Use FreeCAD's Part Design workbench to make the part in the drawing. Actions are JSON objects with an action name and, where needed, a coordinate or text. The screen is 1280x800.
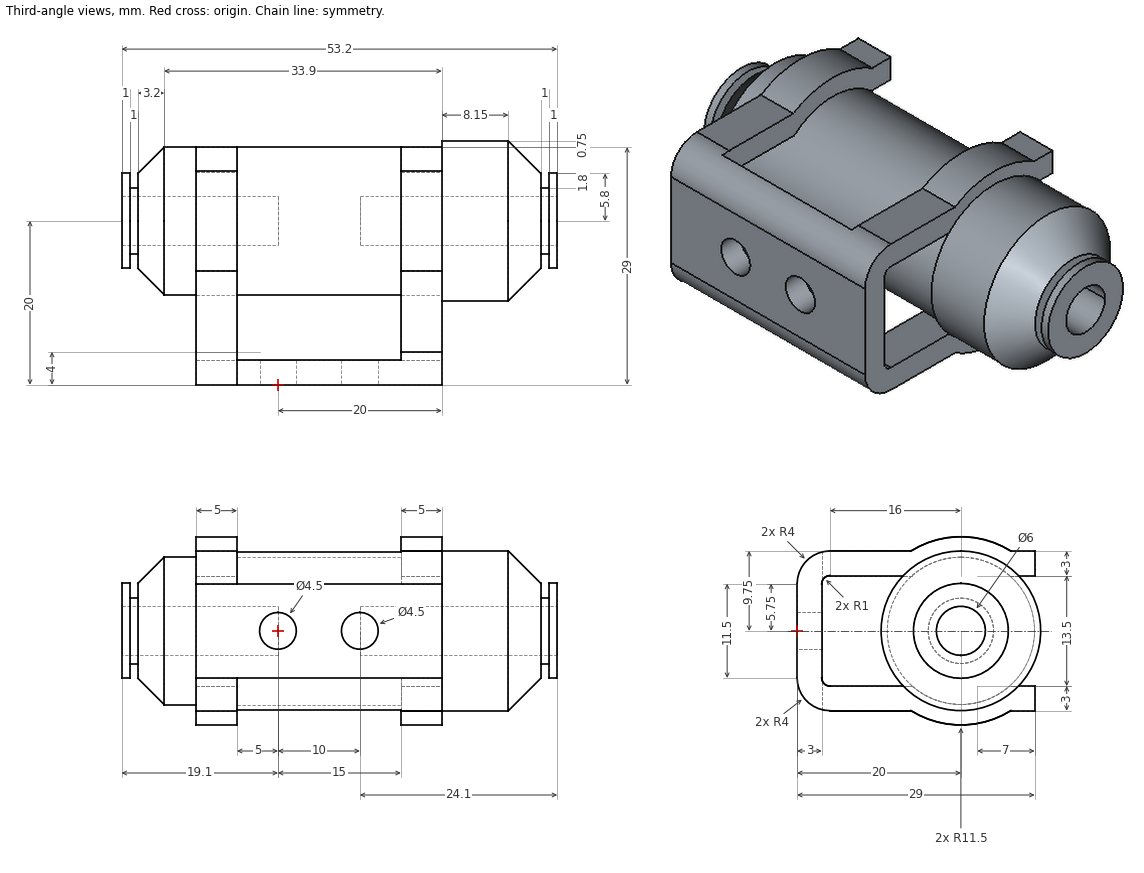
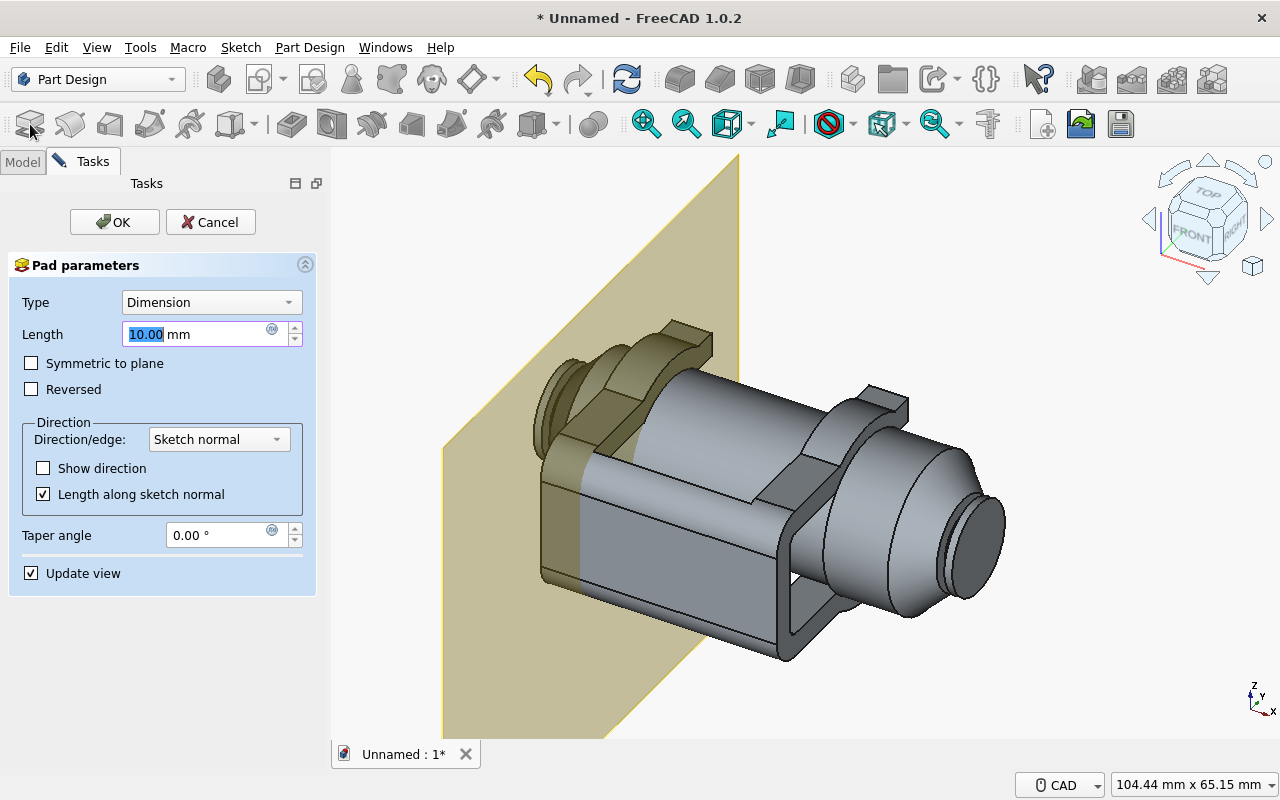
{"action": "type", "text": "5"}
{"action": "key", "text": "Tab"}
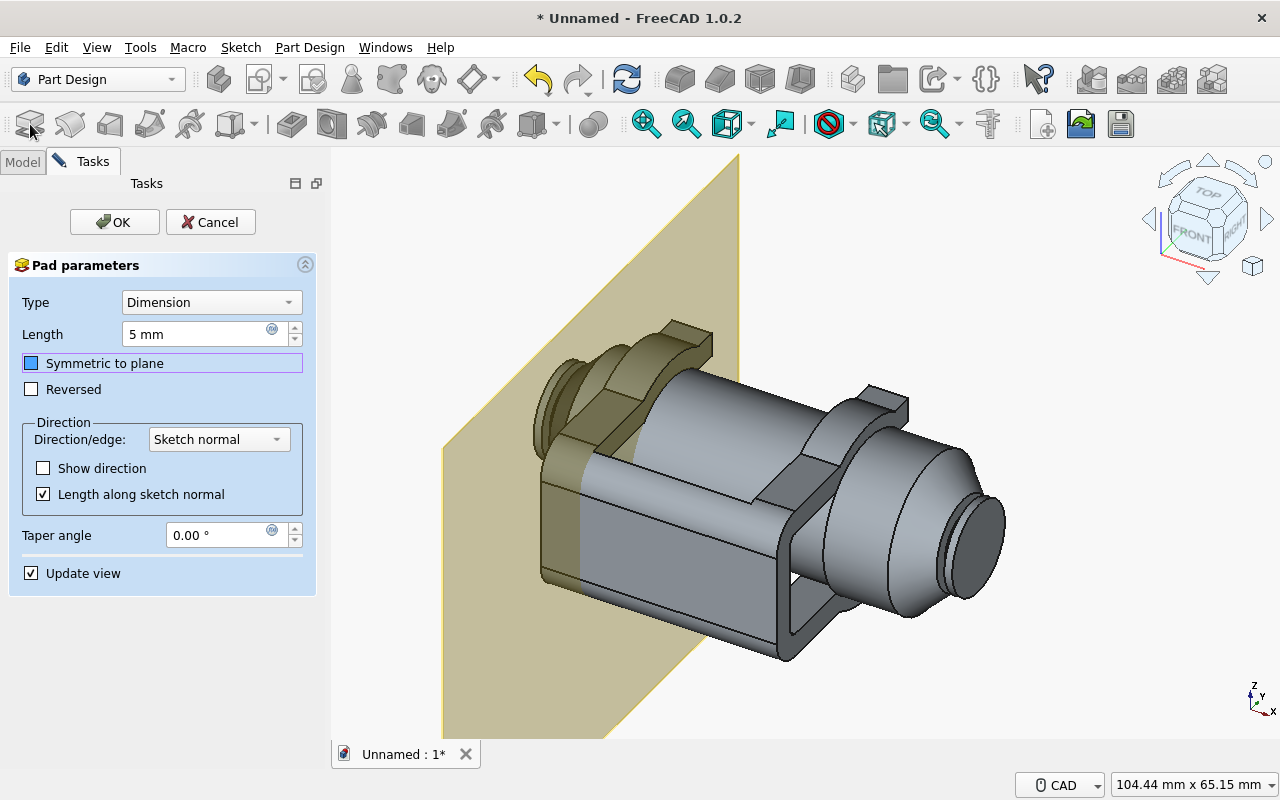
{"action": "left_click", "coordinate": [115, 222]}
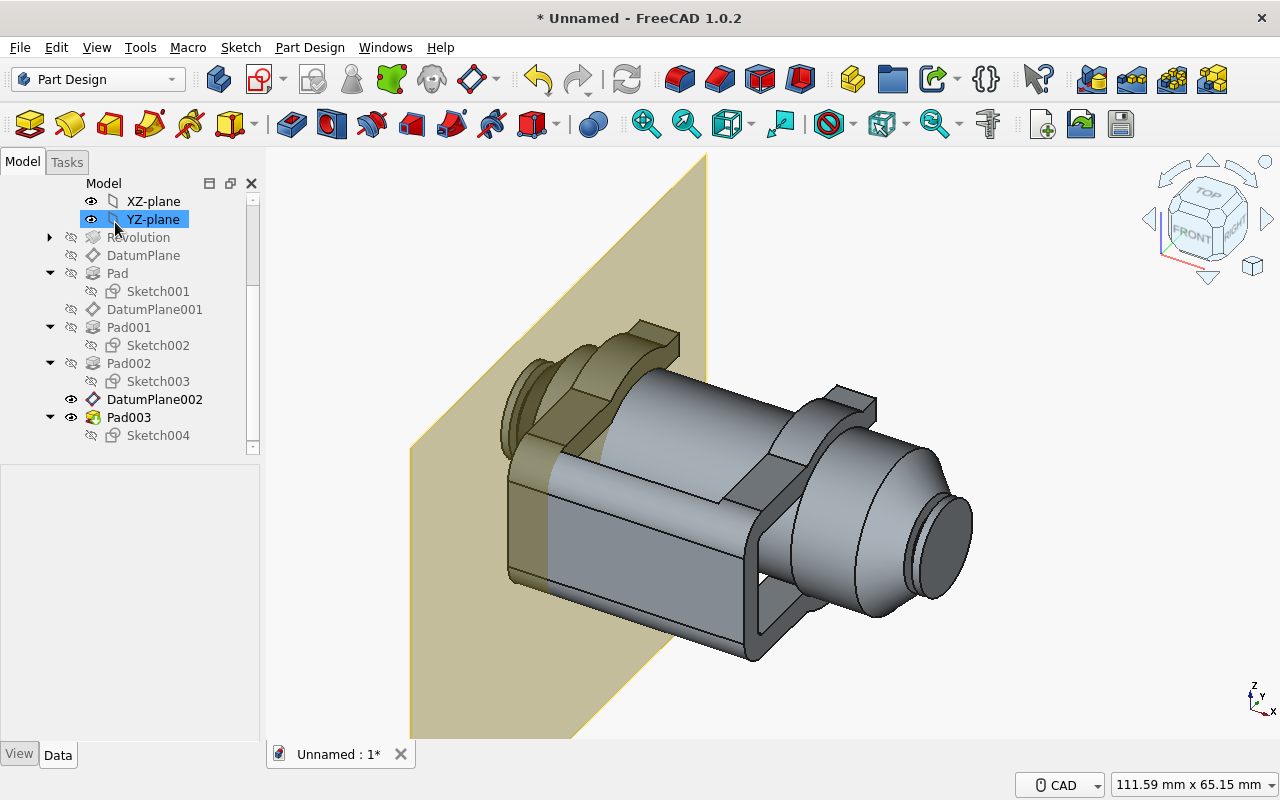
{"action": "left_click", "coordinate": [116, 399]}
{"action": "key", "text": "space"}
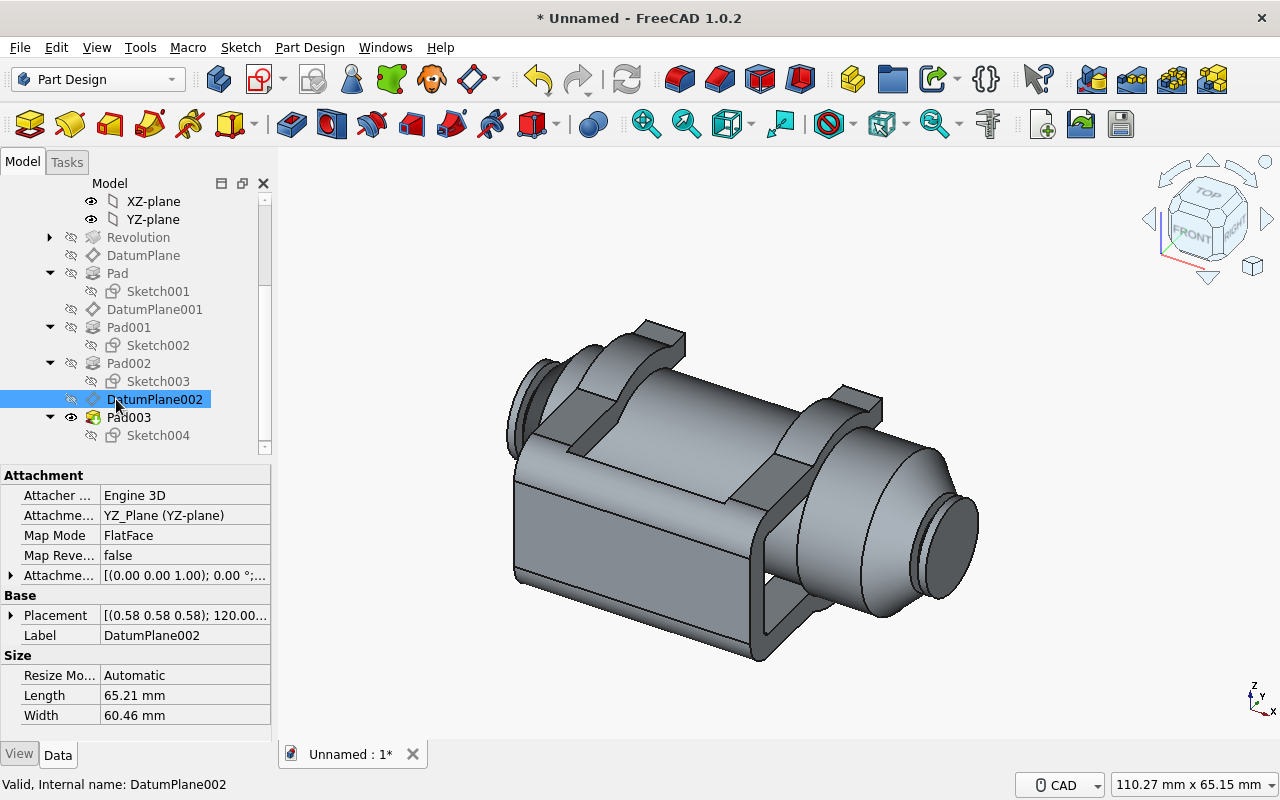
{"action": "left_click", "coordinate": [318, 699]}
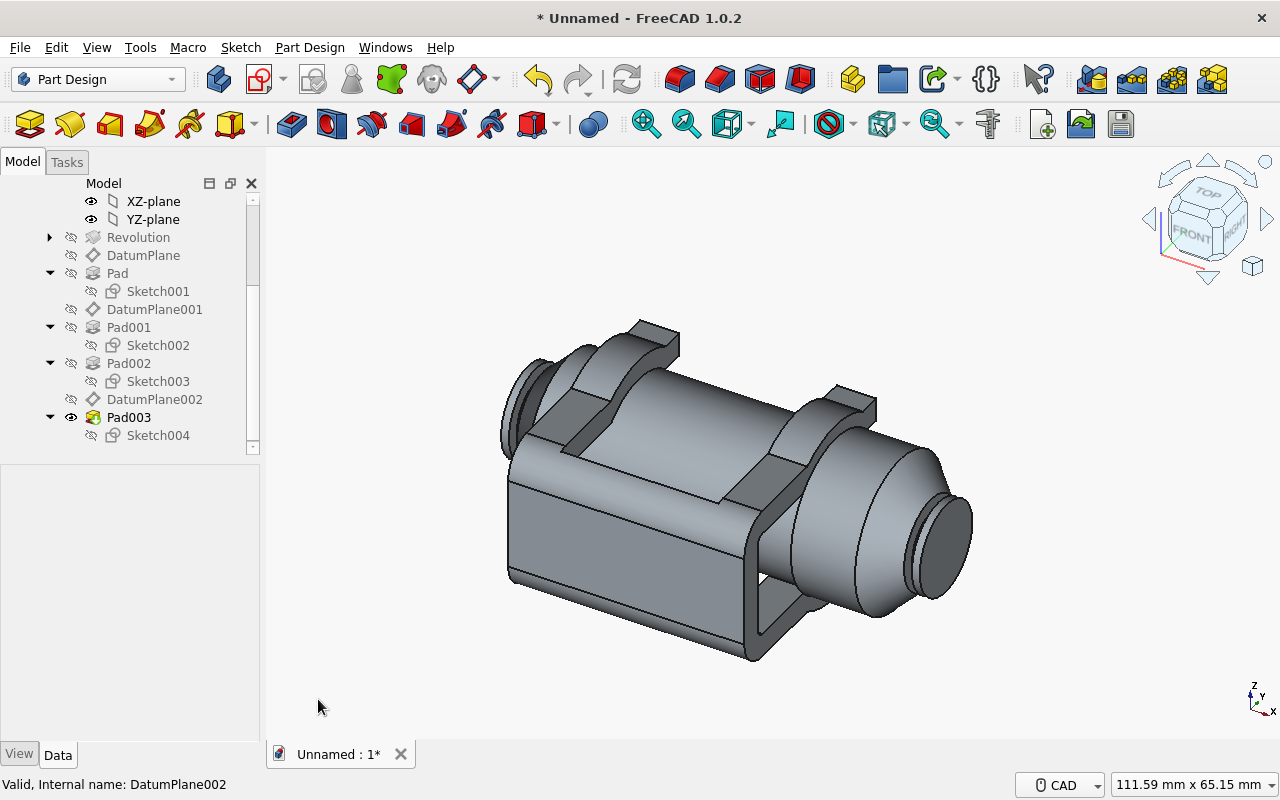
{"action": "left_click", "coordinate": [260, 80]}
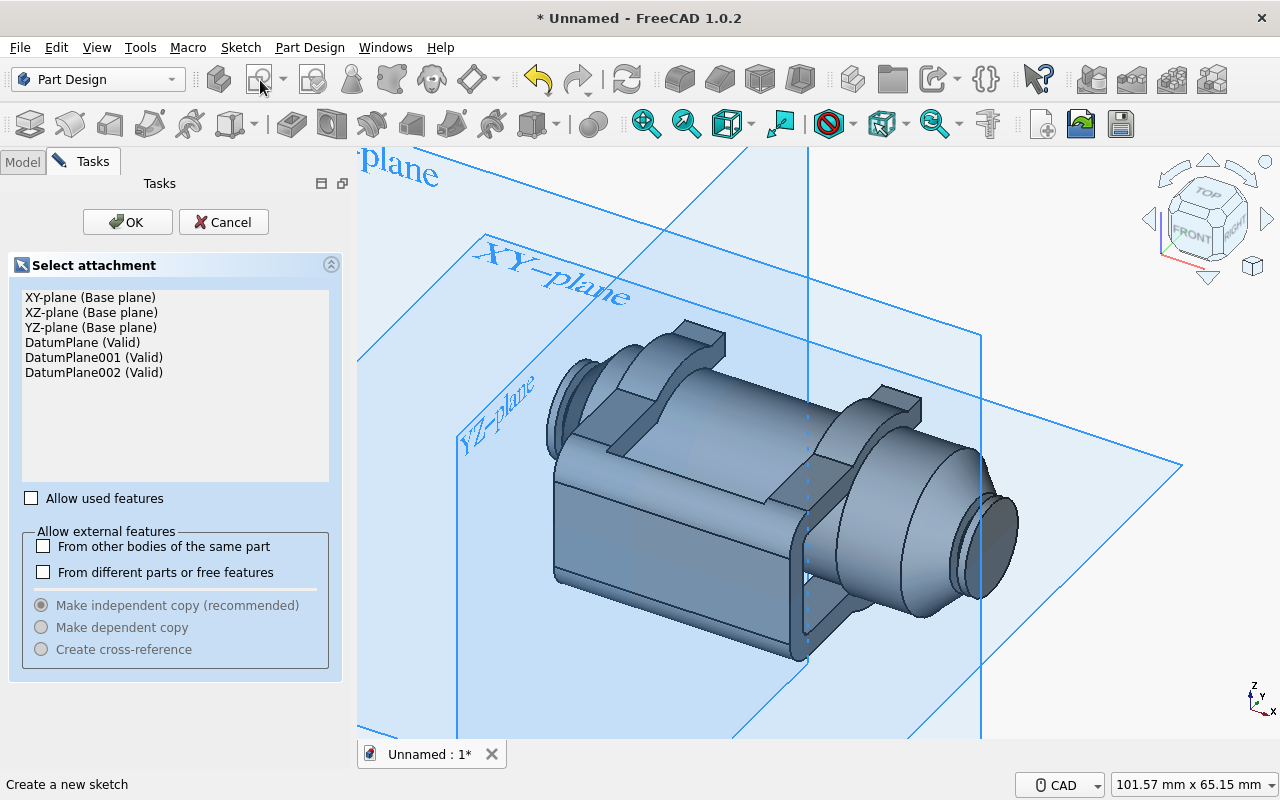
{"action": "left_click", "coordinate": [82, 312]}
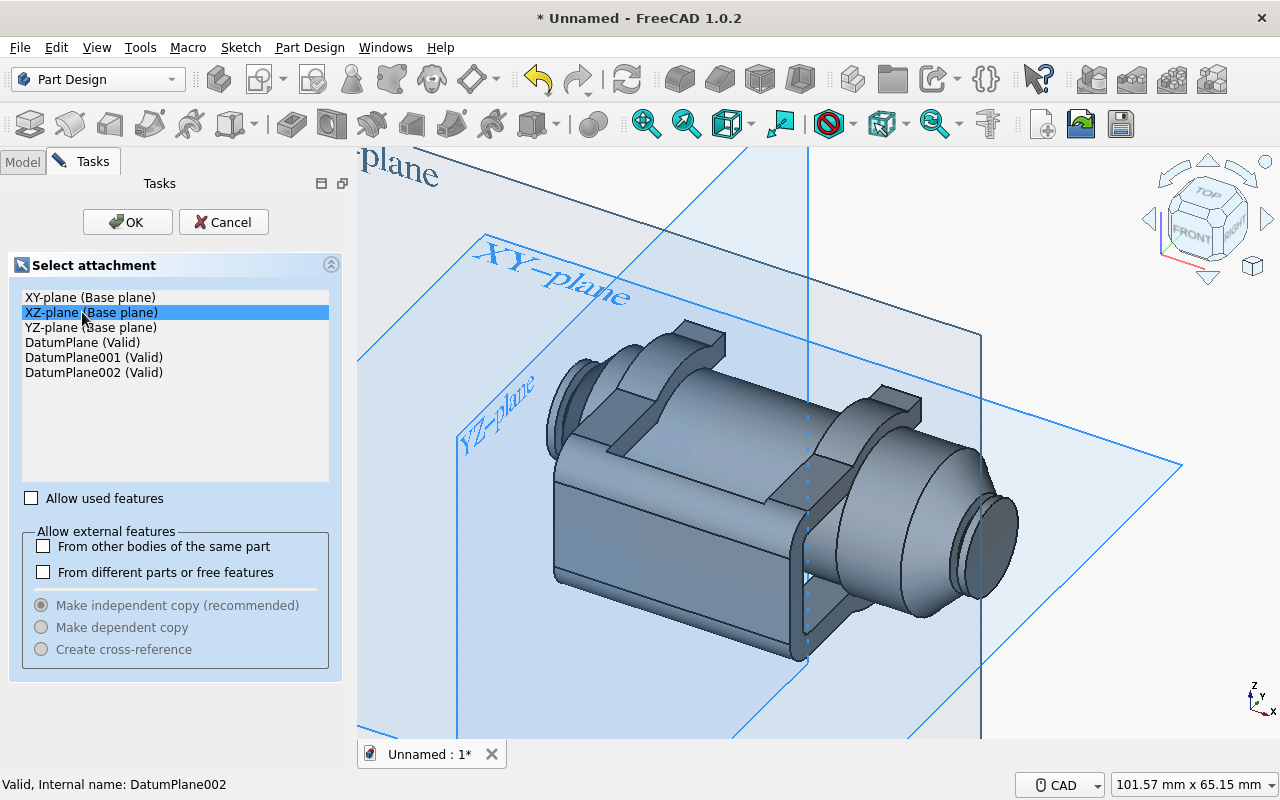
{"action": "left_click", "coordinate": [128, 222]}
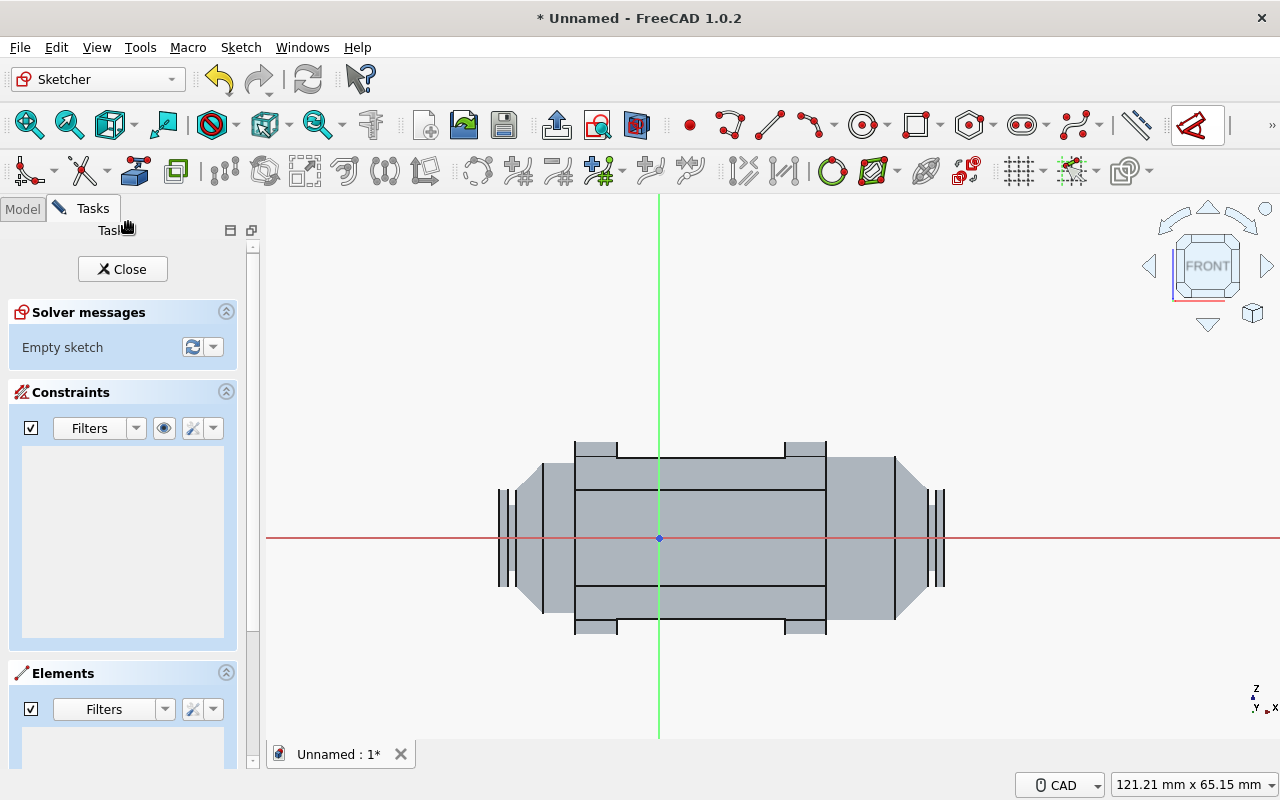
{"action": "scroll", "coordinate": [653, 547], "scroll_direction": "up", "scroll_amount": 11}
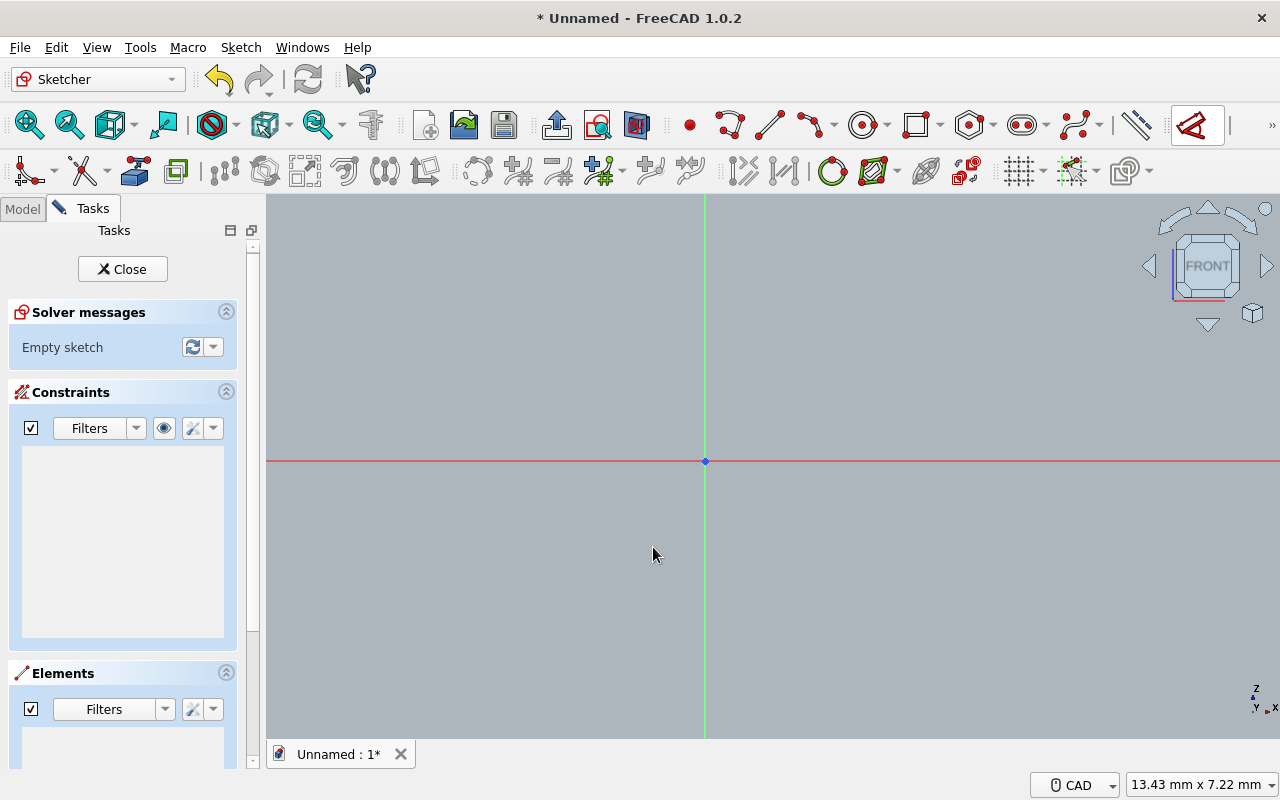
{"action": "left_click", "coordinate": [864, 126]}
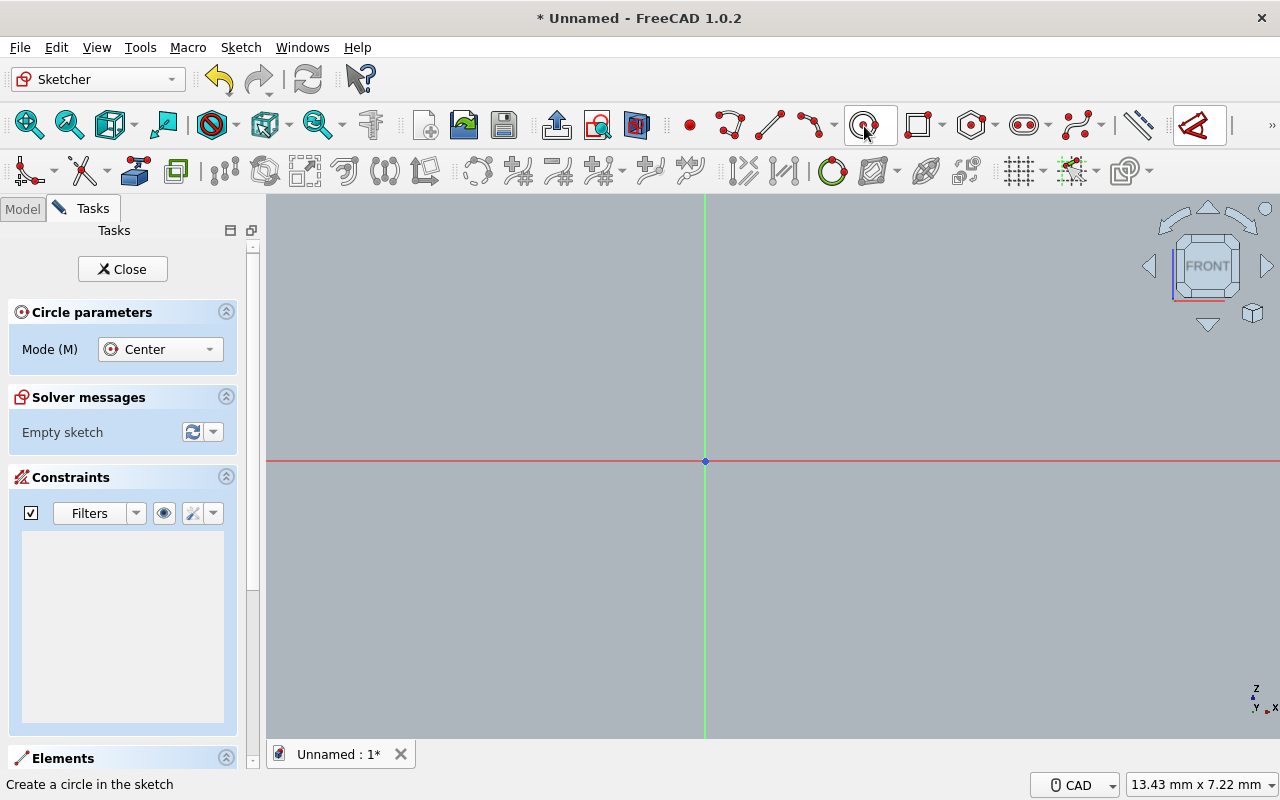
{"action": "left_click", "coordinate": [705, 461]}
{"action": "left_click", "coordinate": [825, 341]}
{"action": "key", "text": "Escape"}